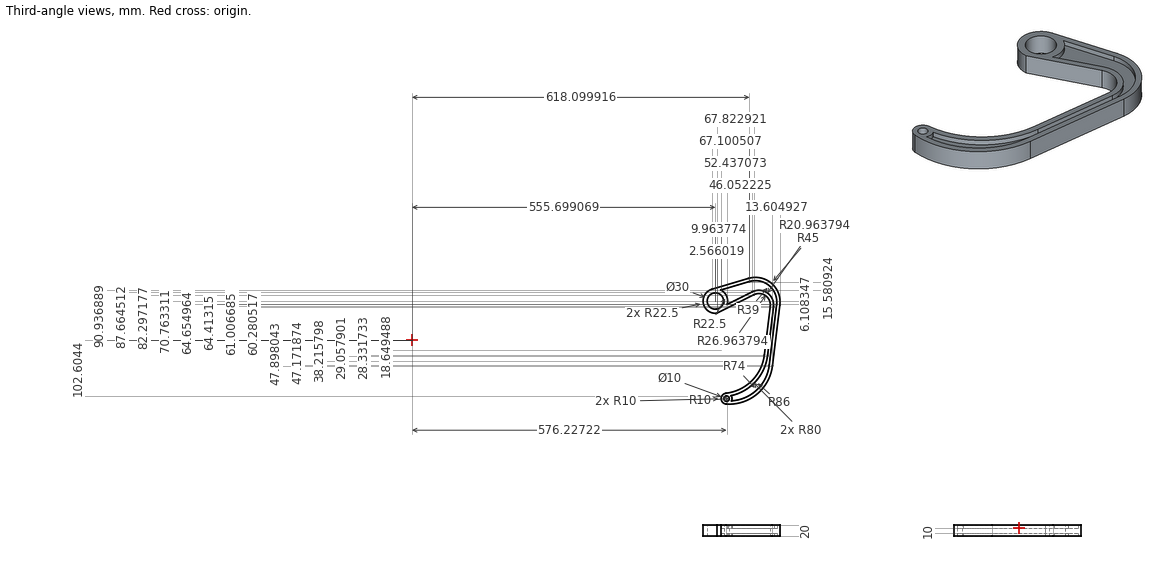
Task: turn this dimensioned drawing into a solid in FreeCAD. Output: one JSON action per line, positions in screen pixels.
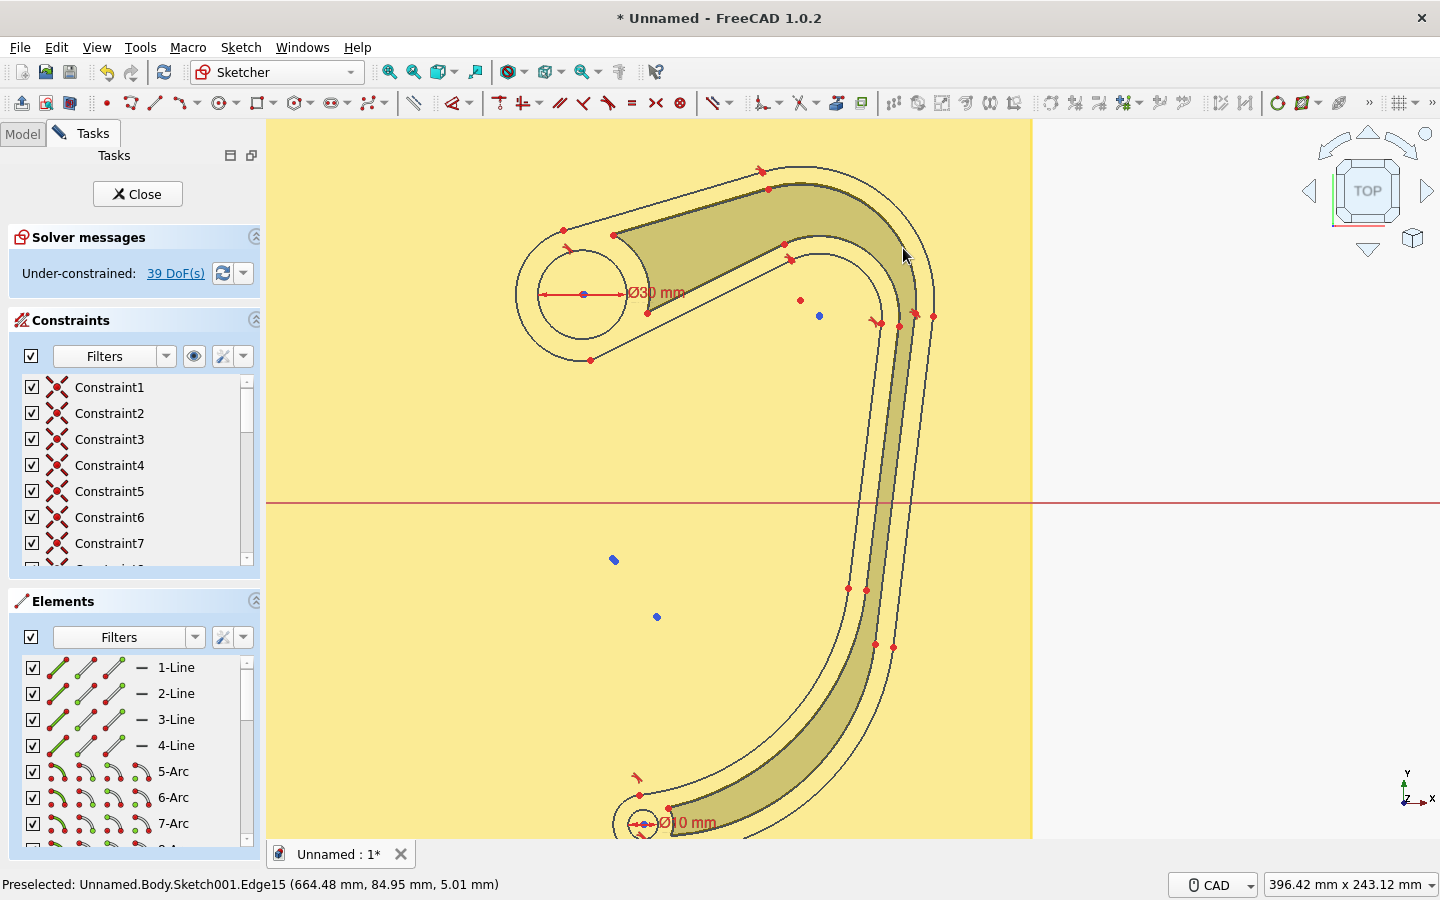
{"action": "left_click", "coordinate": [856, 747]}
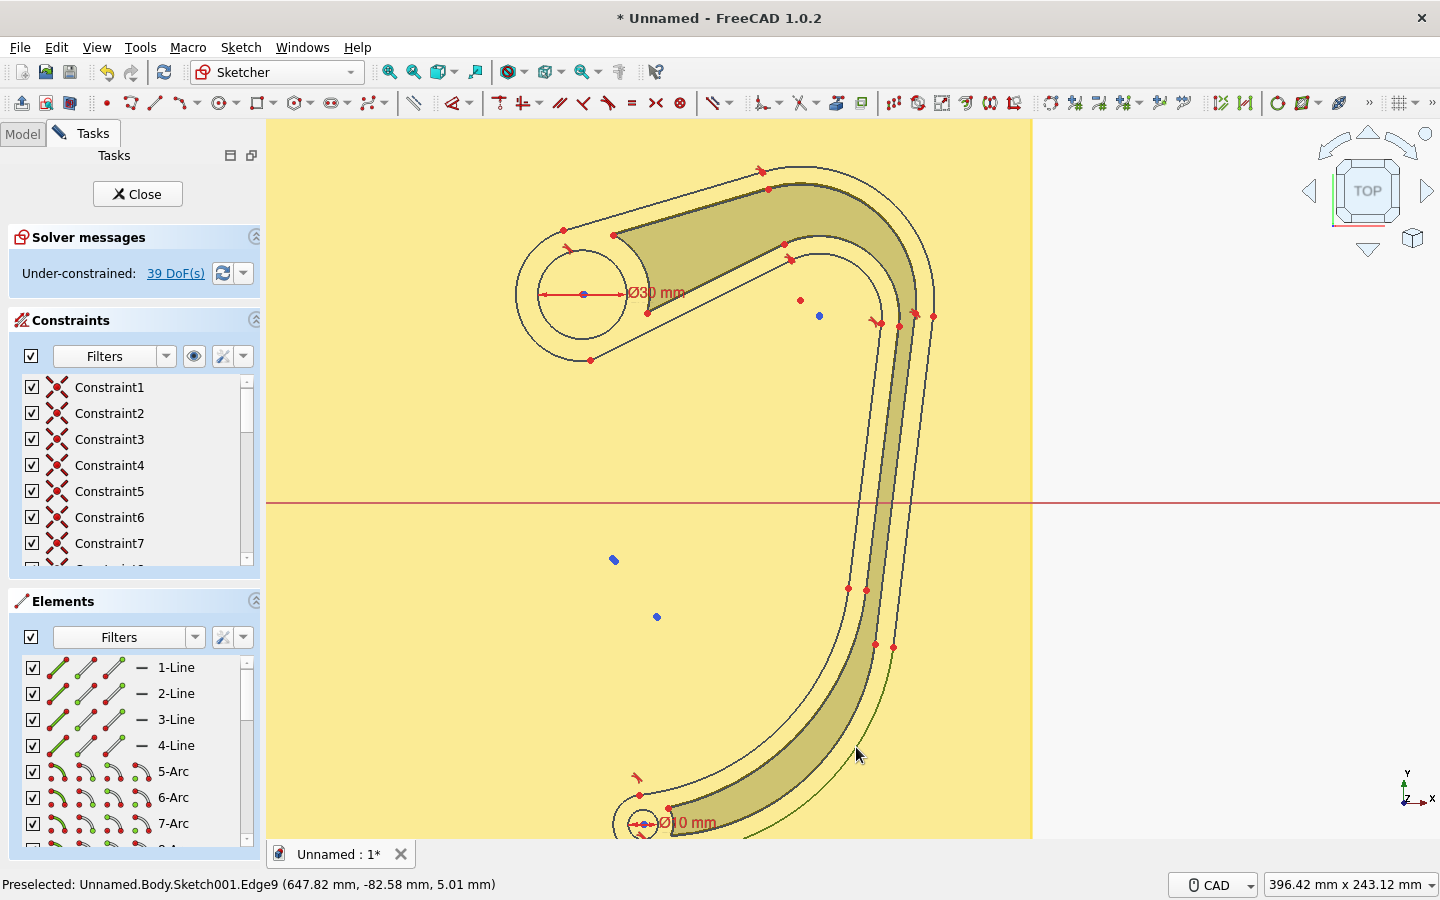
{"action": "left_click", "coordinate": [846, 730]}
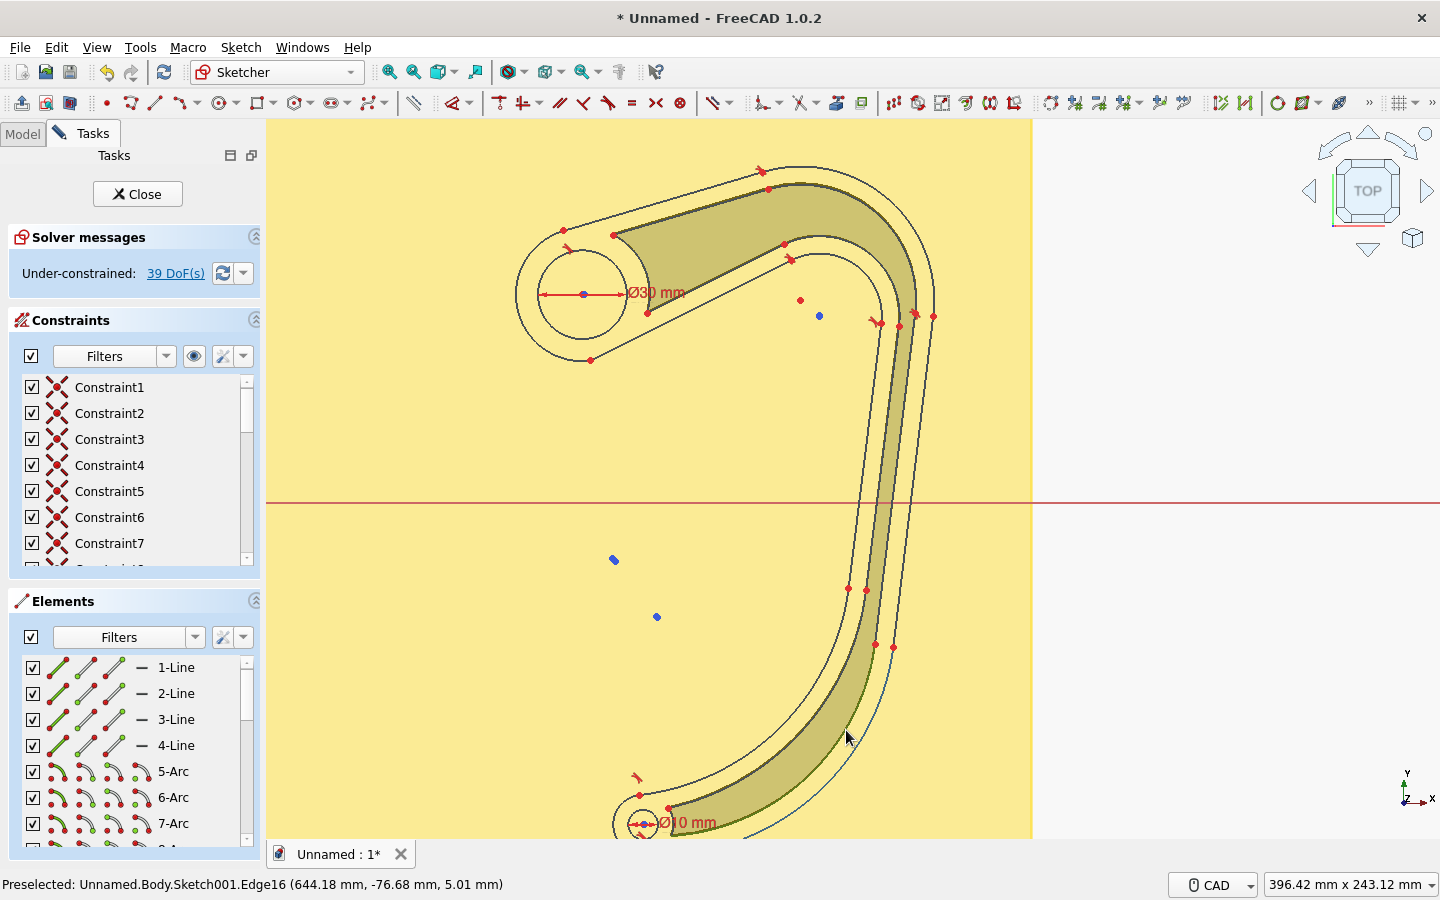
{"action": "left_click", "coordinate": [500, 104]}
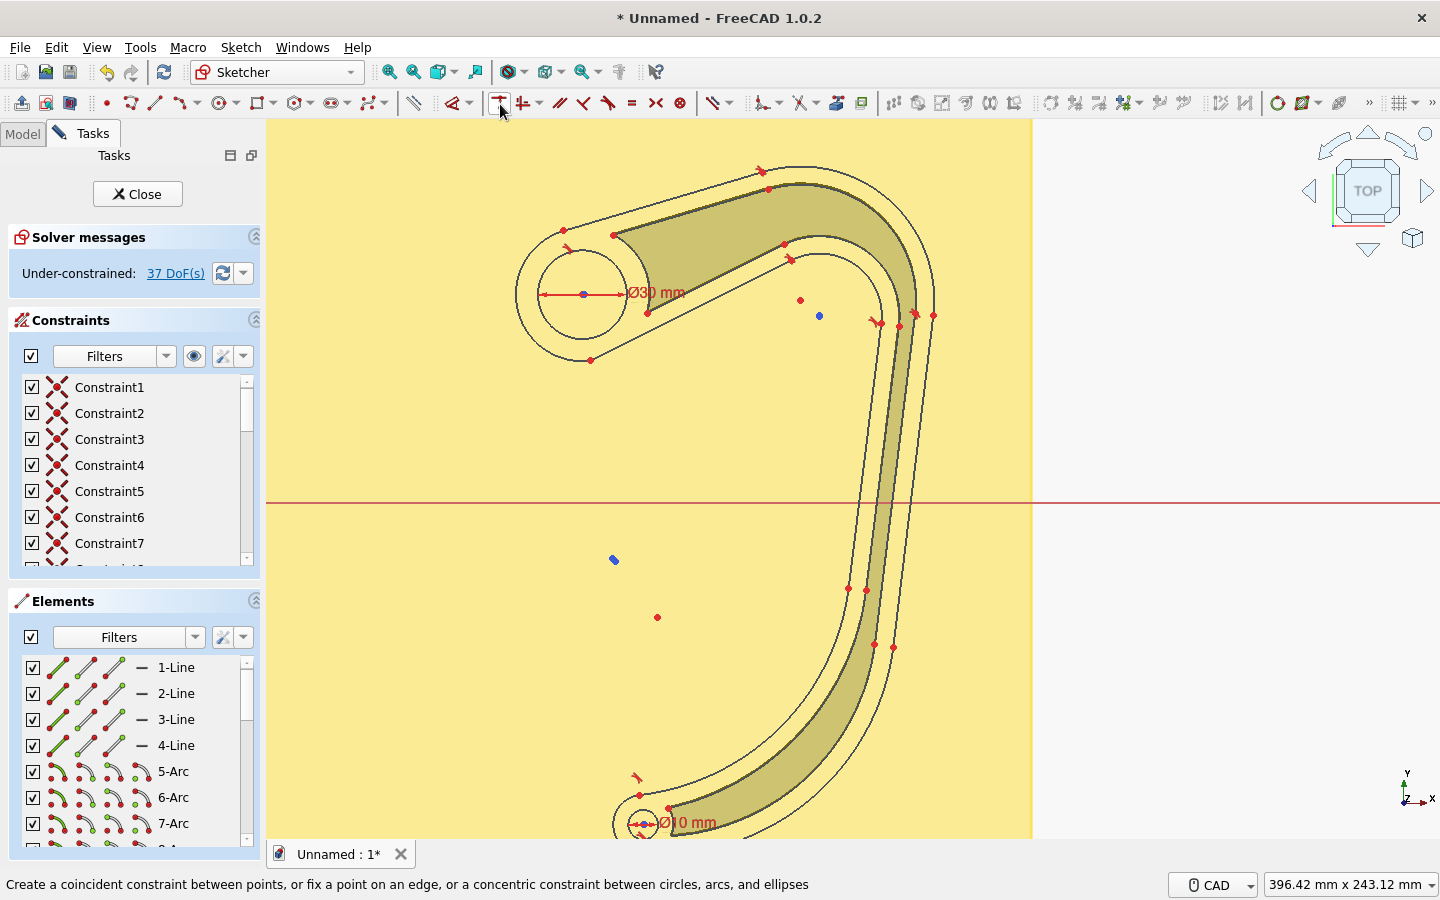
{"action": "left_click", "coordinate": [644, 810]}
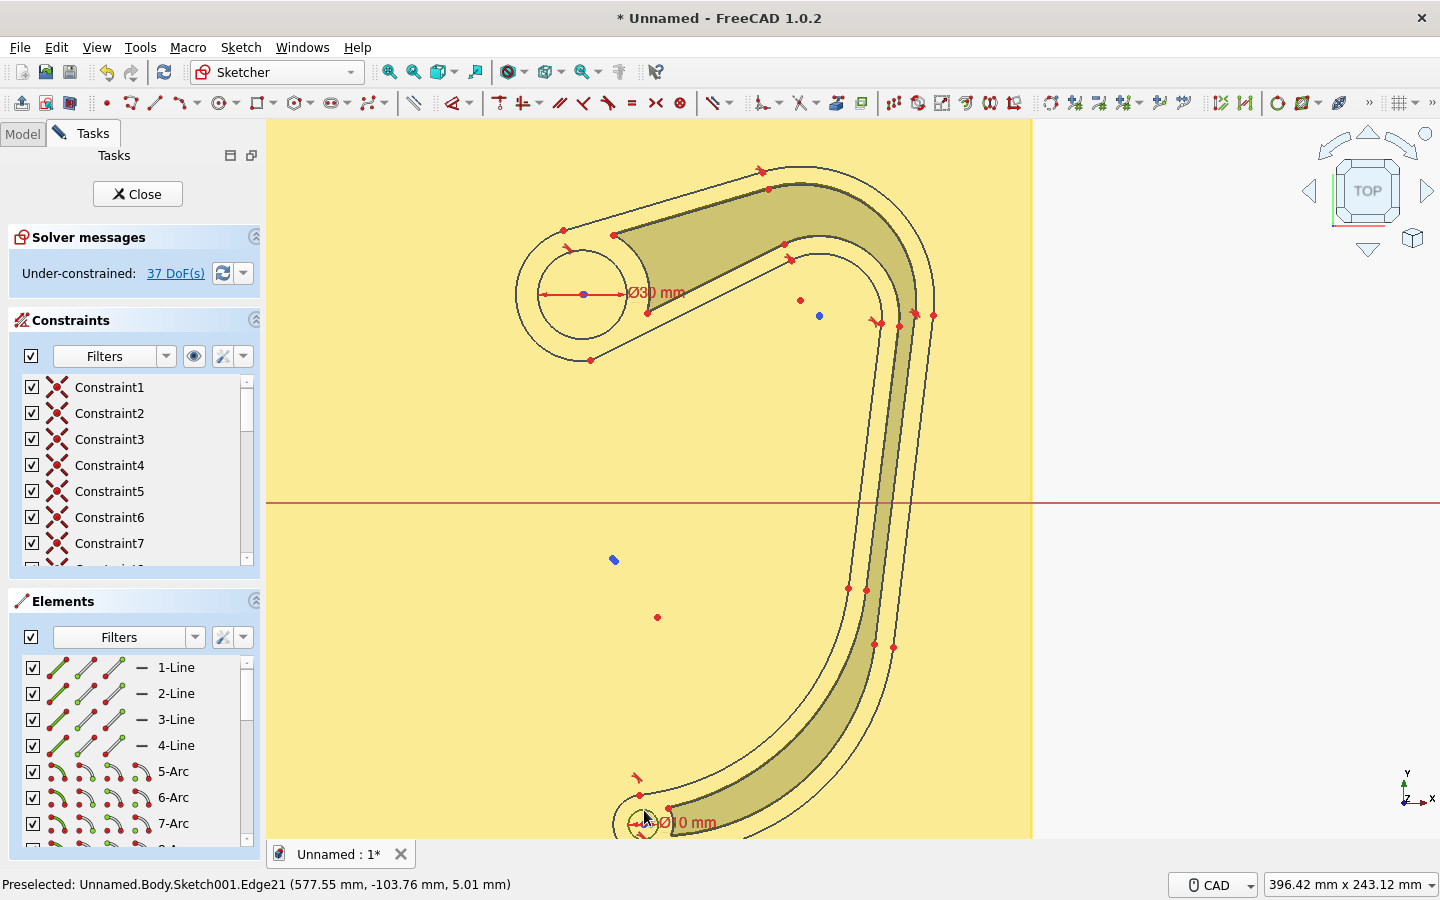
{"action": "scroll", "coordinate": [905, 412], "scroll_direction": "down", "scroll_amount": 2}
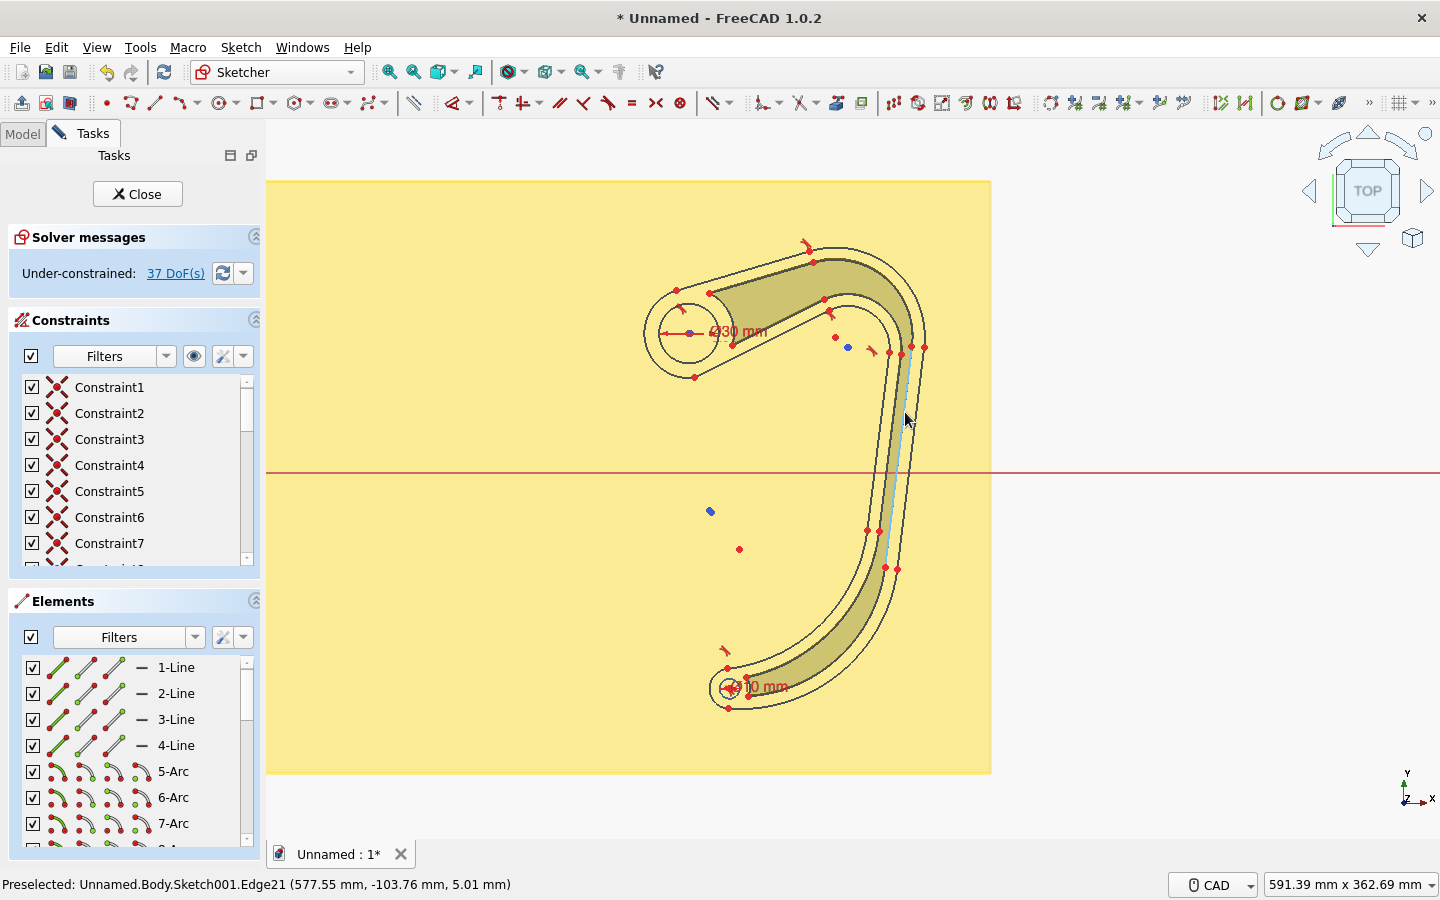
{"action": "scroll", "coordinate": [750, 687], "scroll_direction": "up", "scroll_amount": 2}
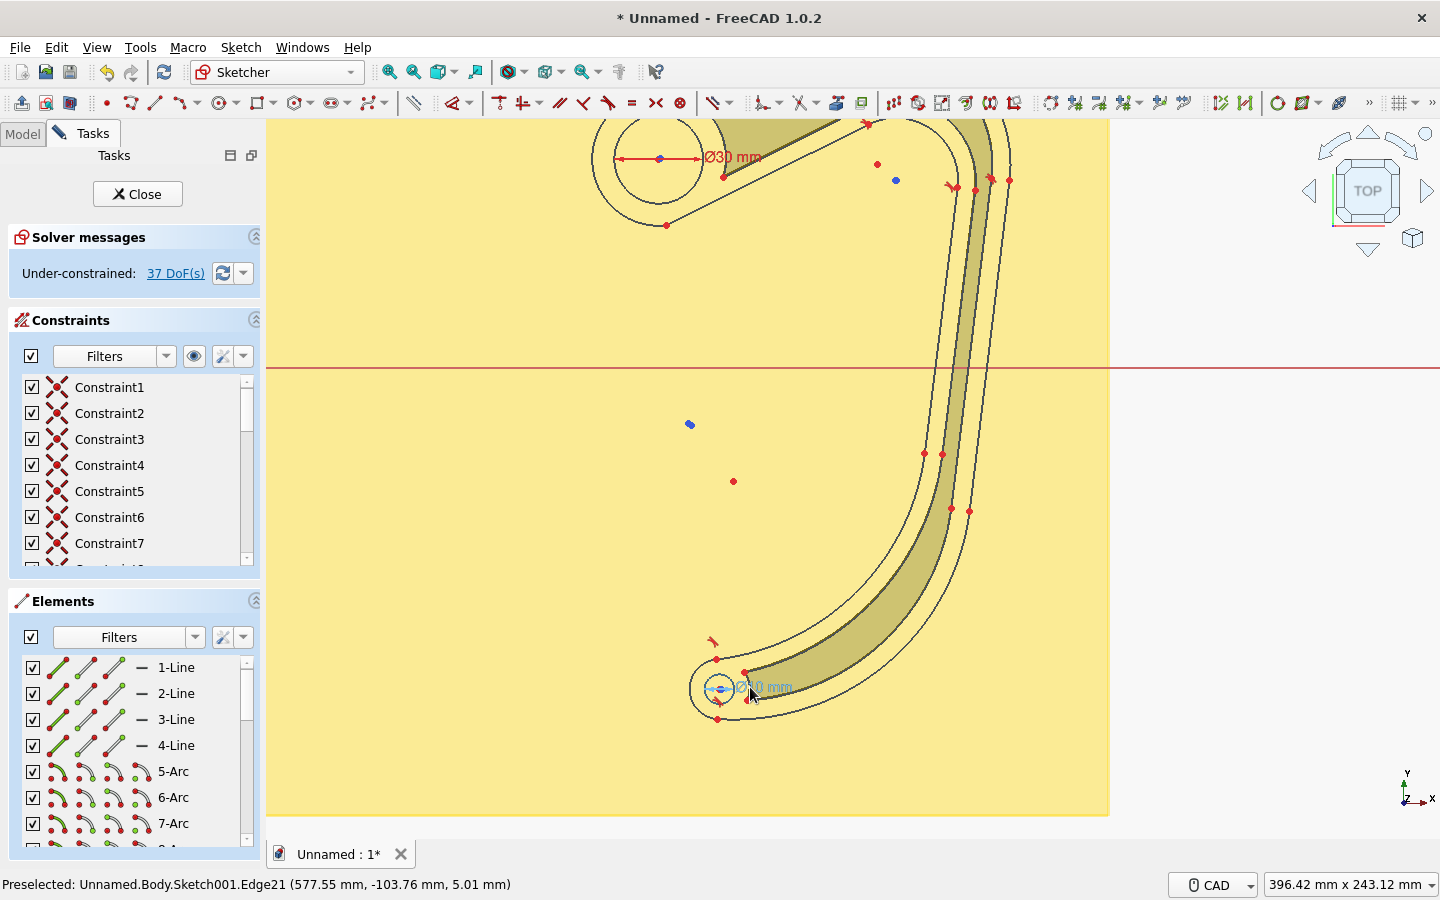
{"action": "left_click", "coordinate": [748, 680]}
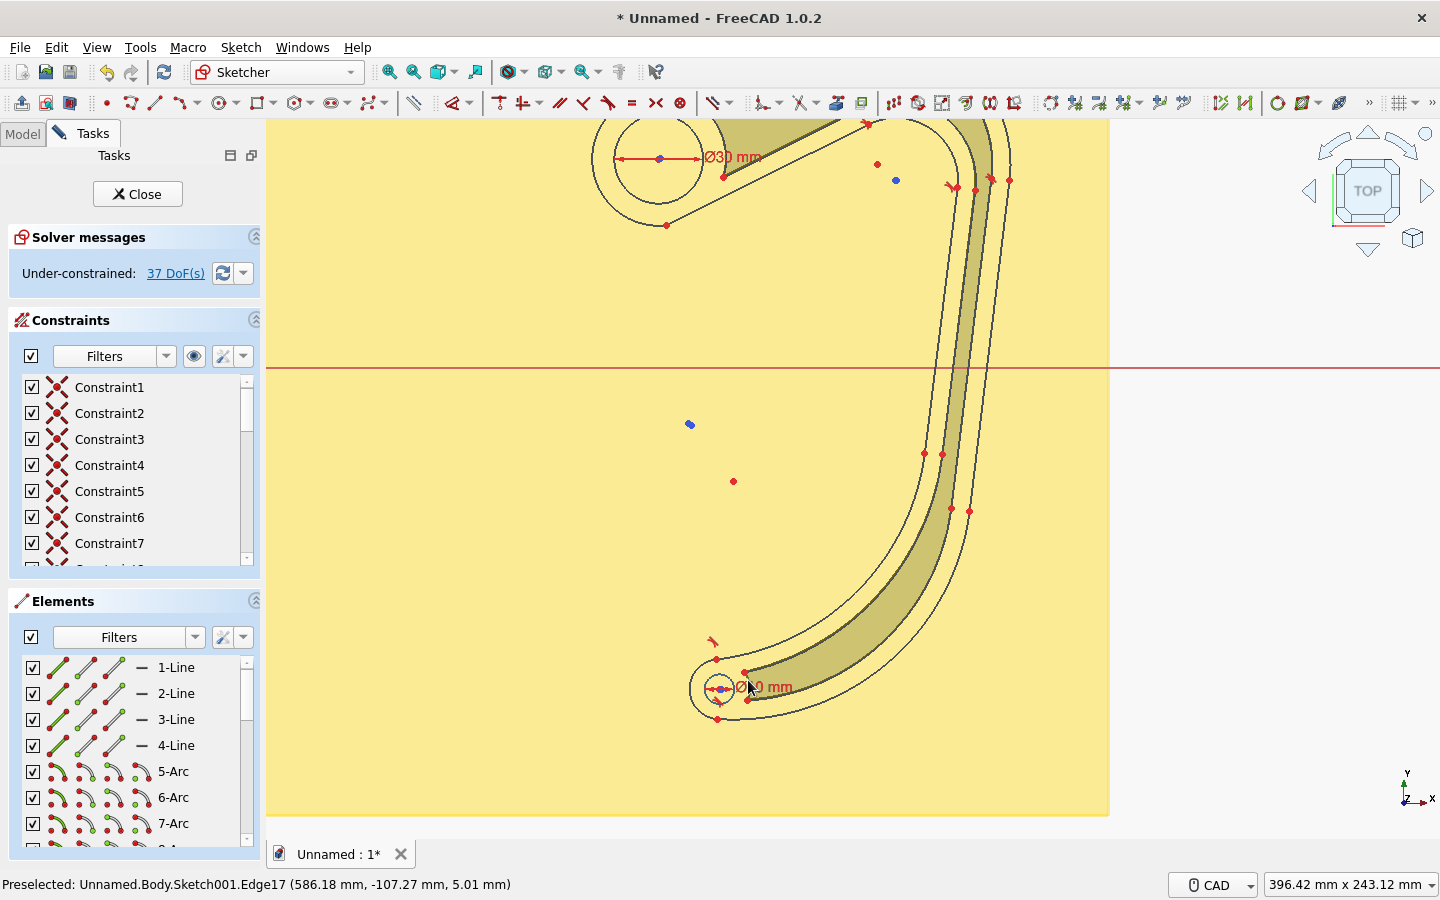
{"action": "left_click", "coordinate": [500, 104]}